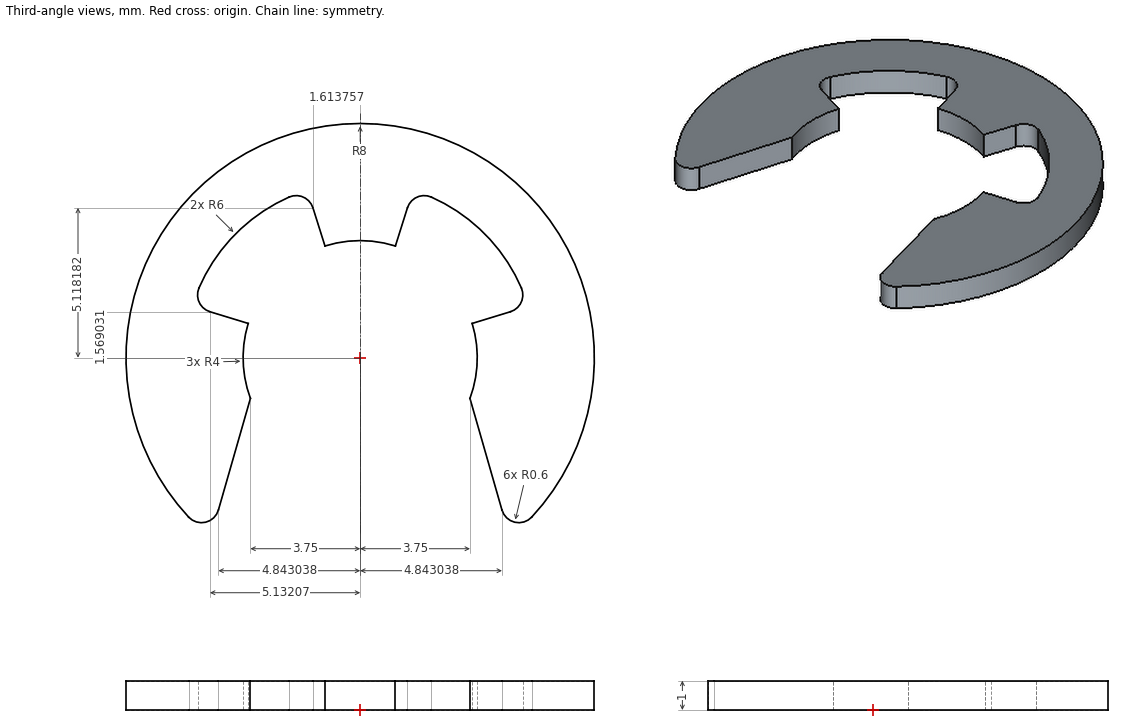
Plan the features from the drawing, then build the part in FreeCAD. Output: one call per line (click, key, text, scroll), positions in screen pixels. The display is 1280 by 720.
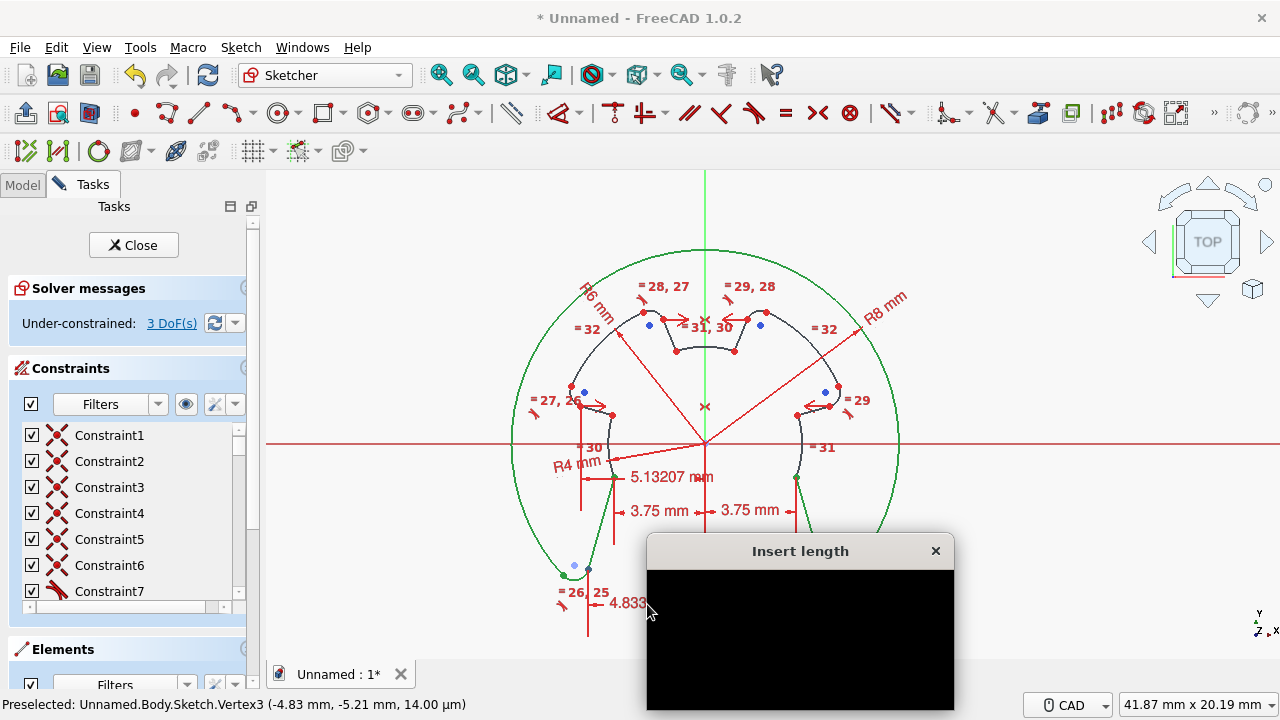
text(4.843038)
key(Return)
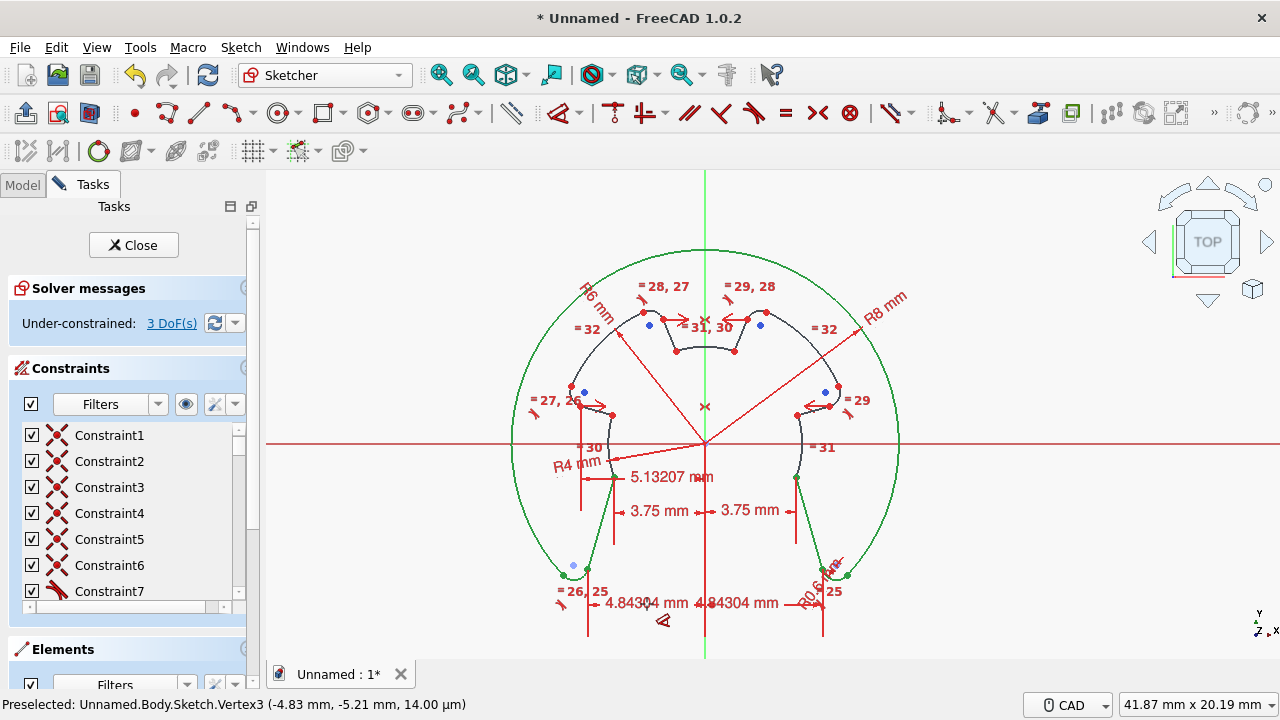
click(581, 406)
click(547, 425)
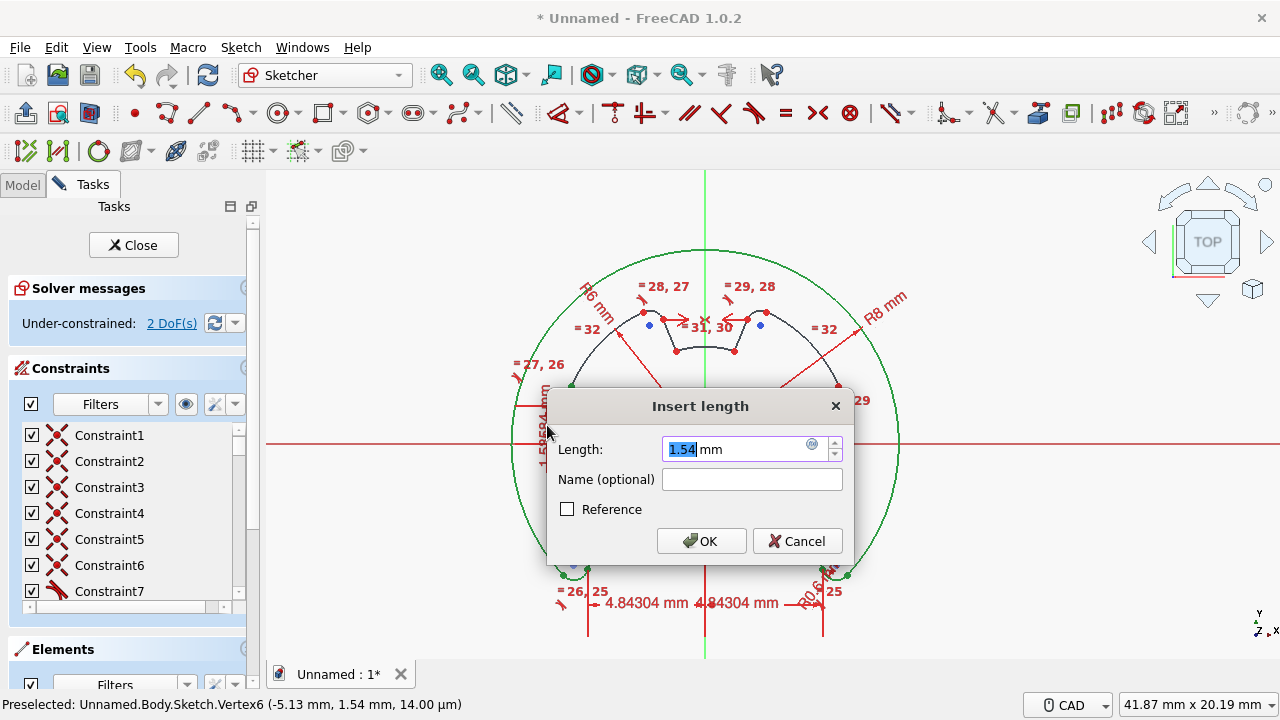
text(1.569031)
key(Return)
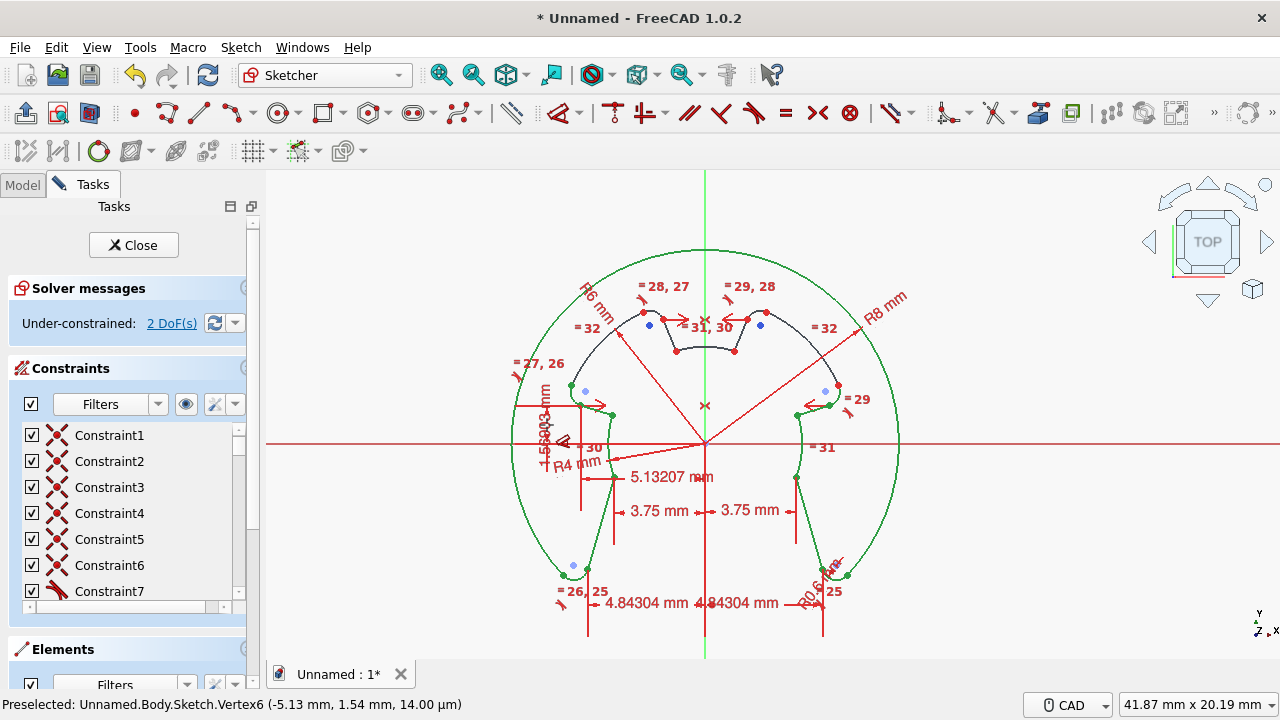
click(663, 320)
click(684, 286)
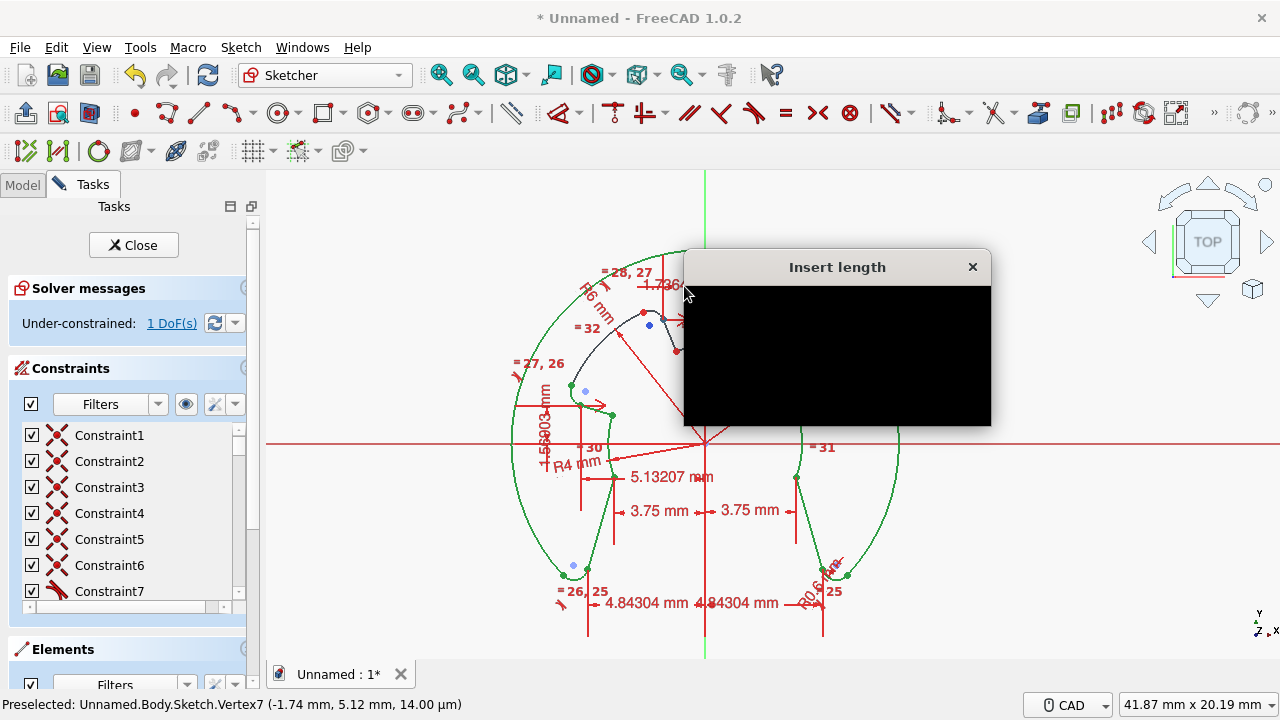
text(1.613757)
key(Return)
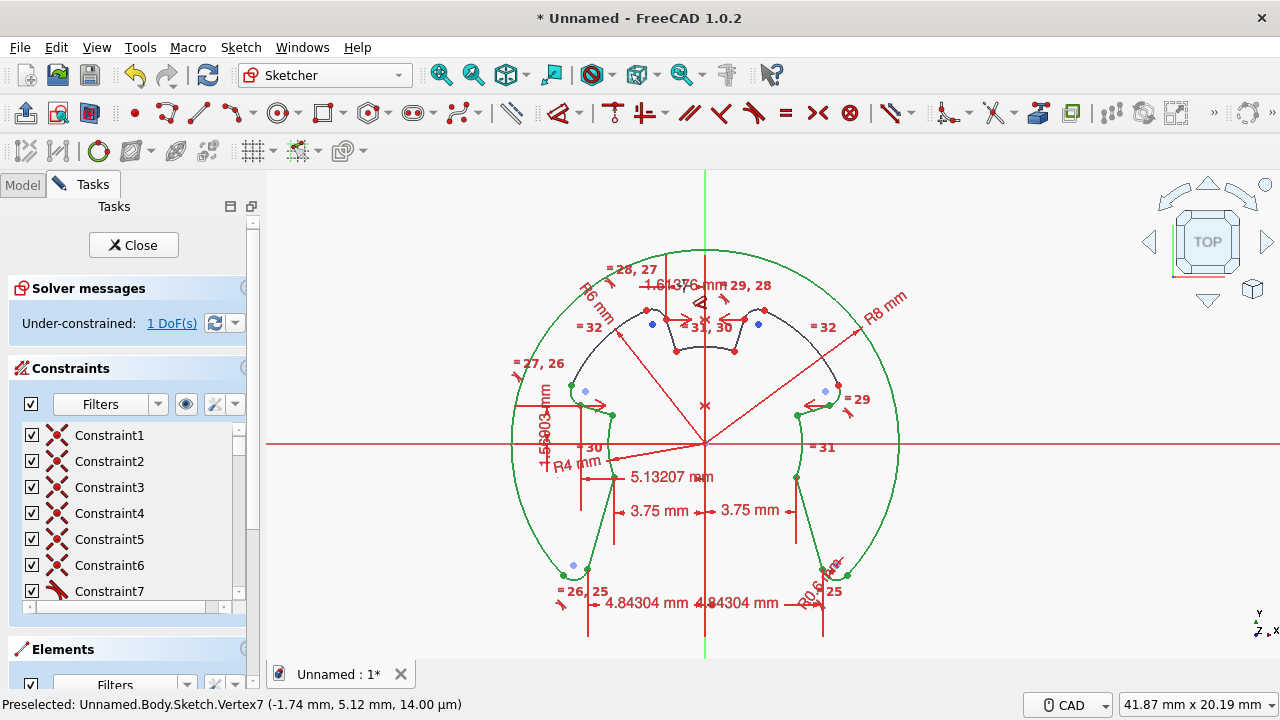
click(666, 320)
click(632, 382)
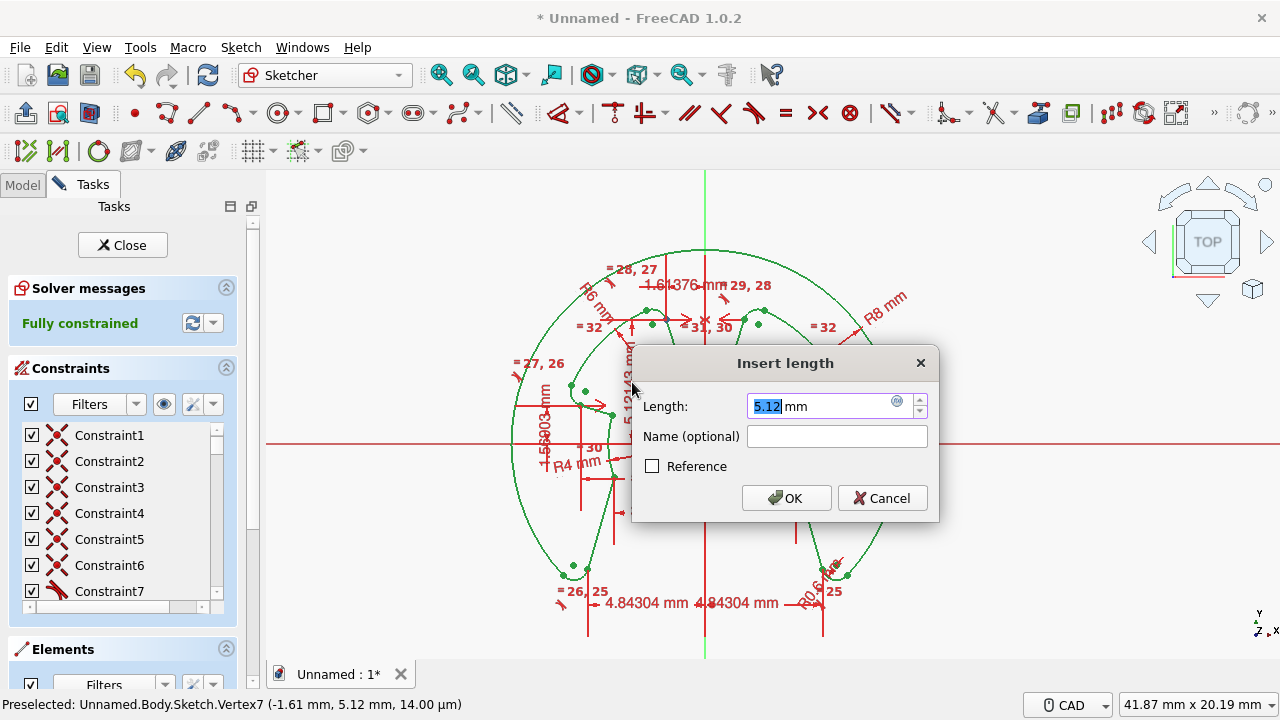
text(5.118182)
key(Return)
key(Escape)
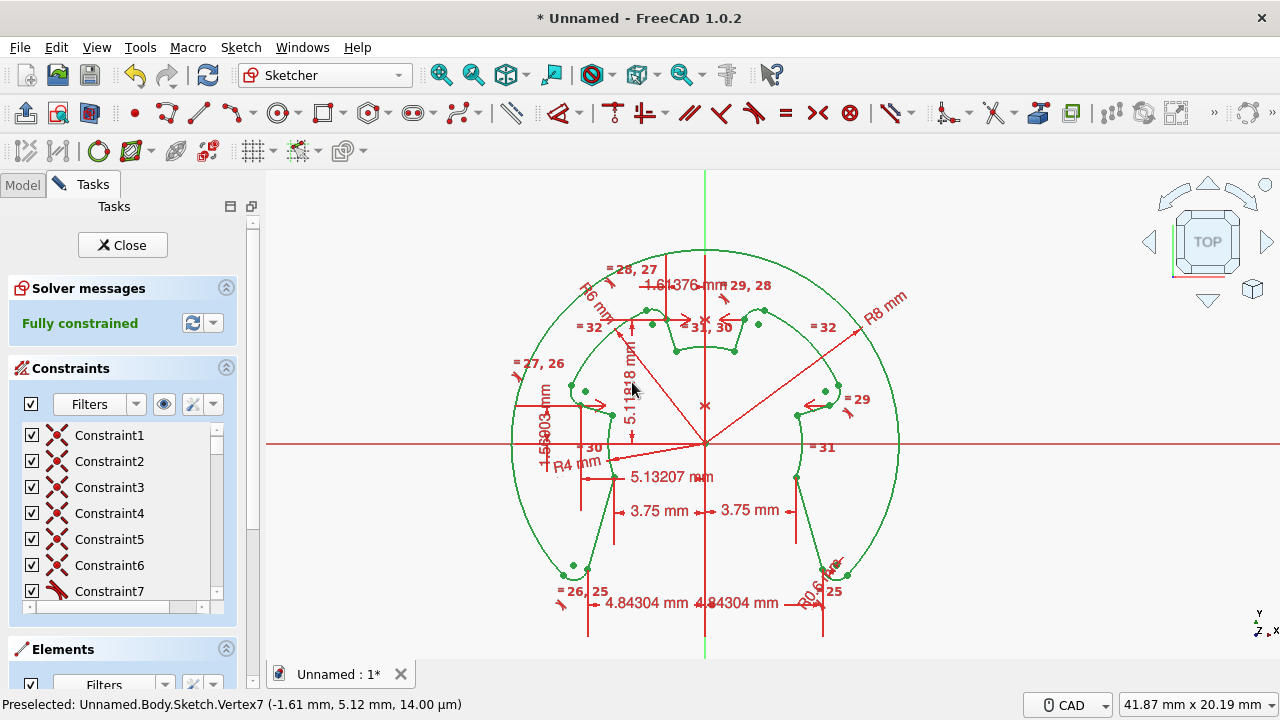
click(123, 245)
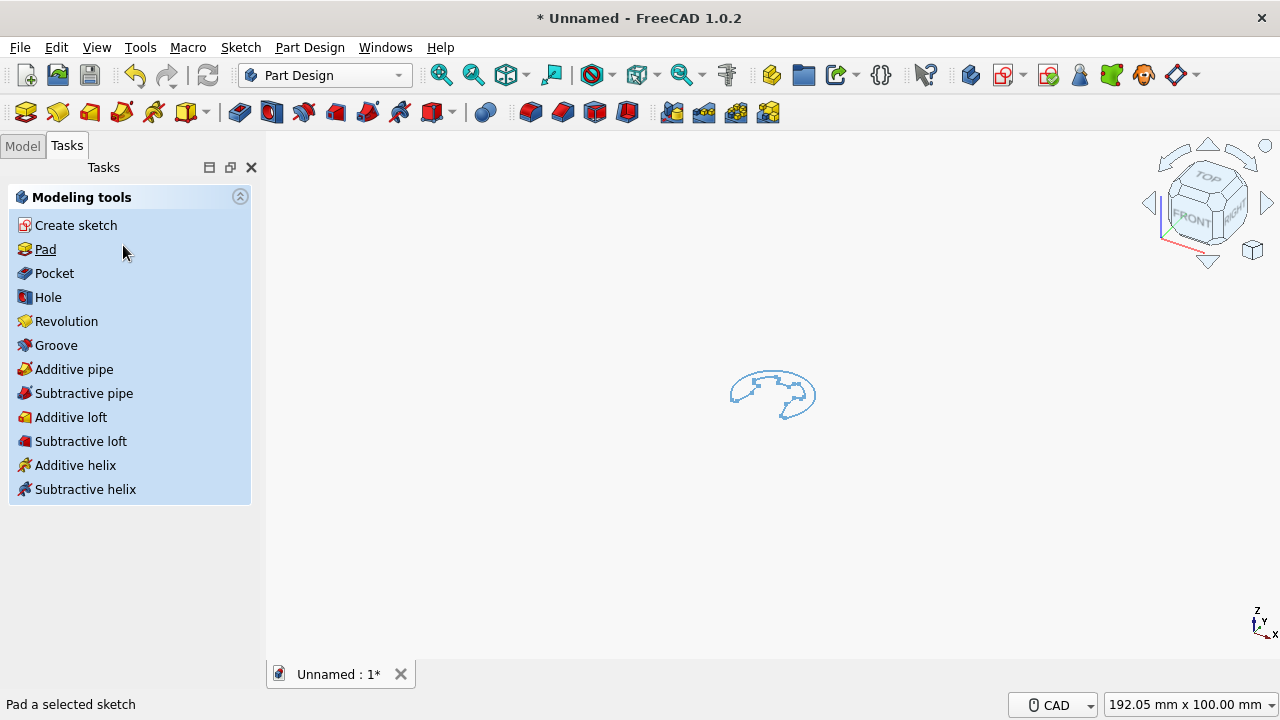
click(26, 112)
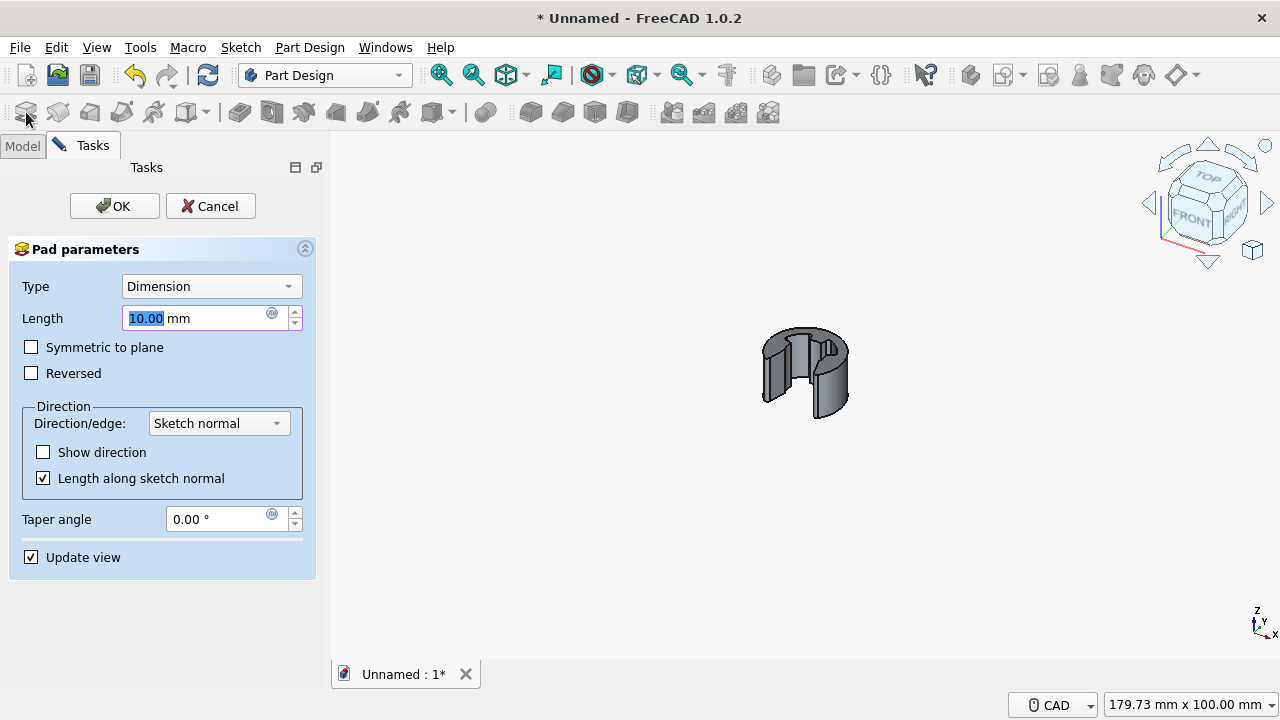
text(1)
key(Tab)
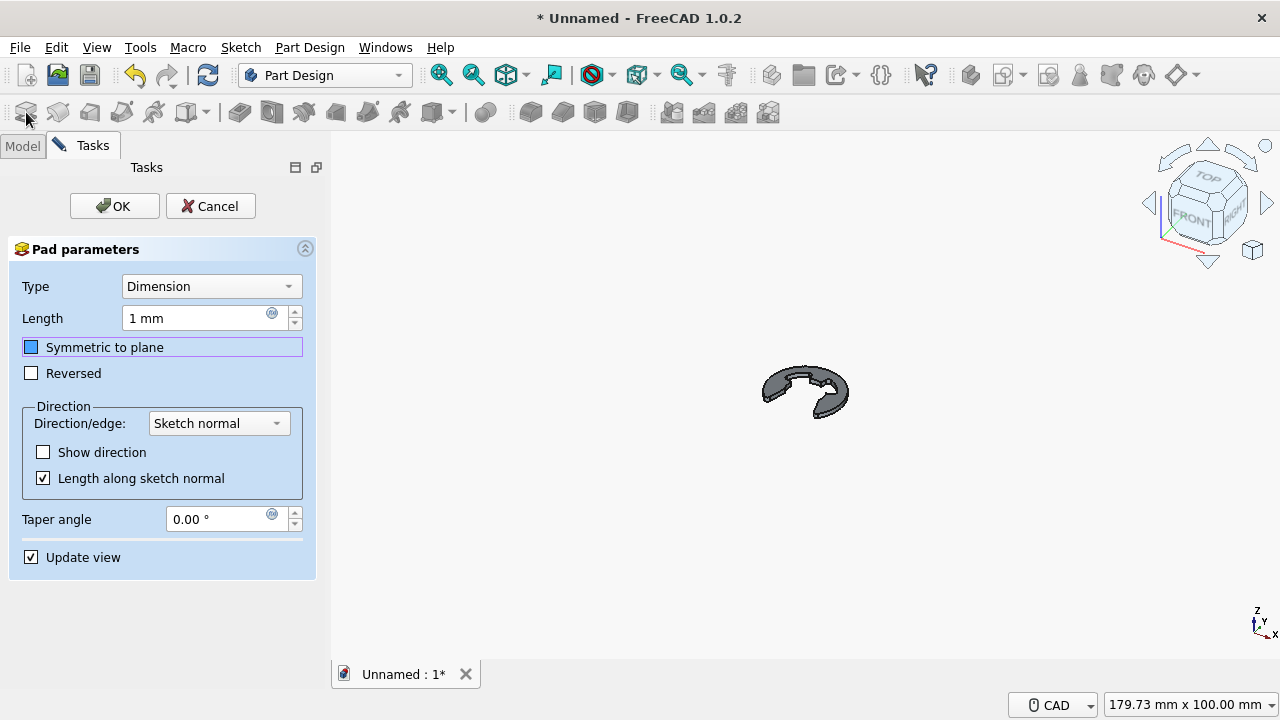
click(115, 206)